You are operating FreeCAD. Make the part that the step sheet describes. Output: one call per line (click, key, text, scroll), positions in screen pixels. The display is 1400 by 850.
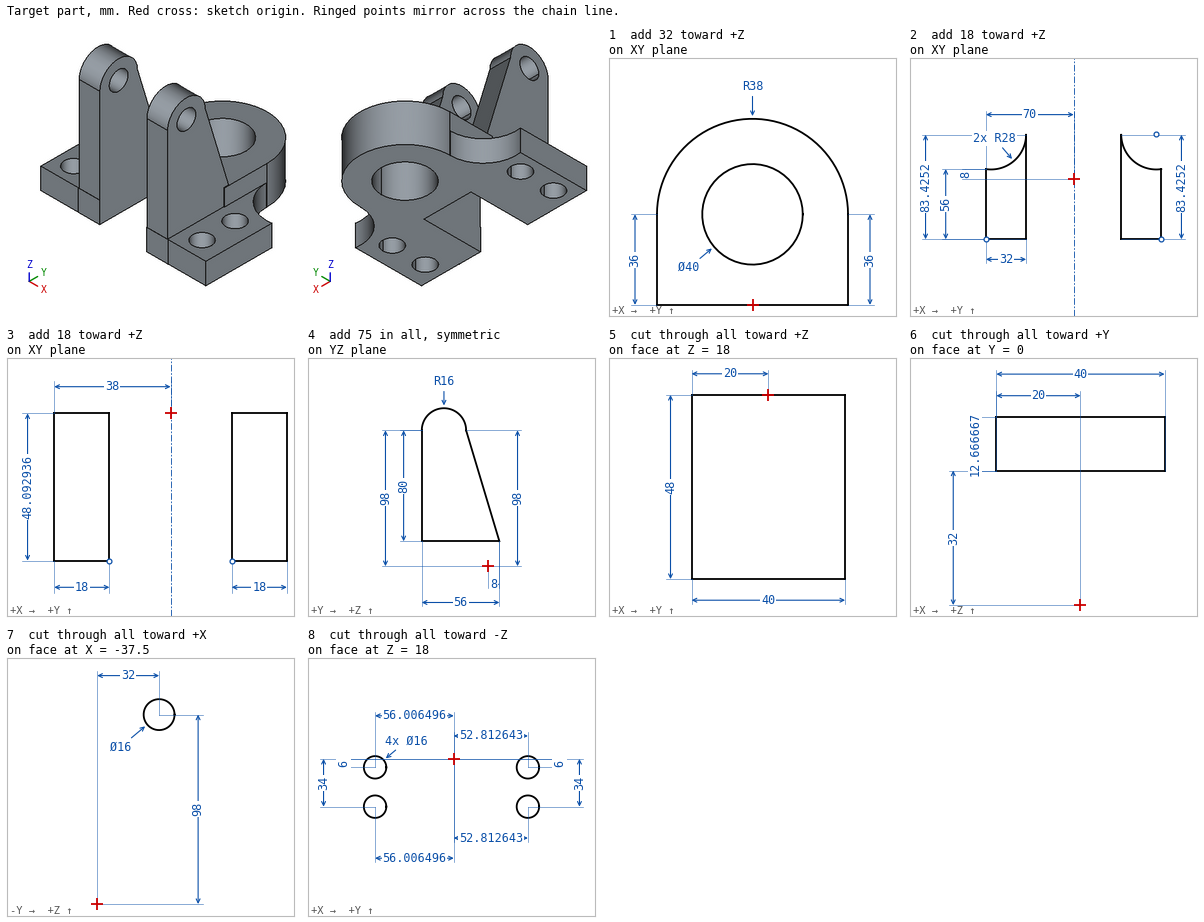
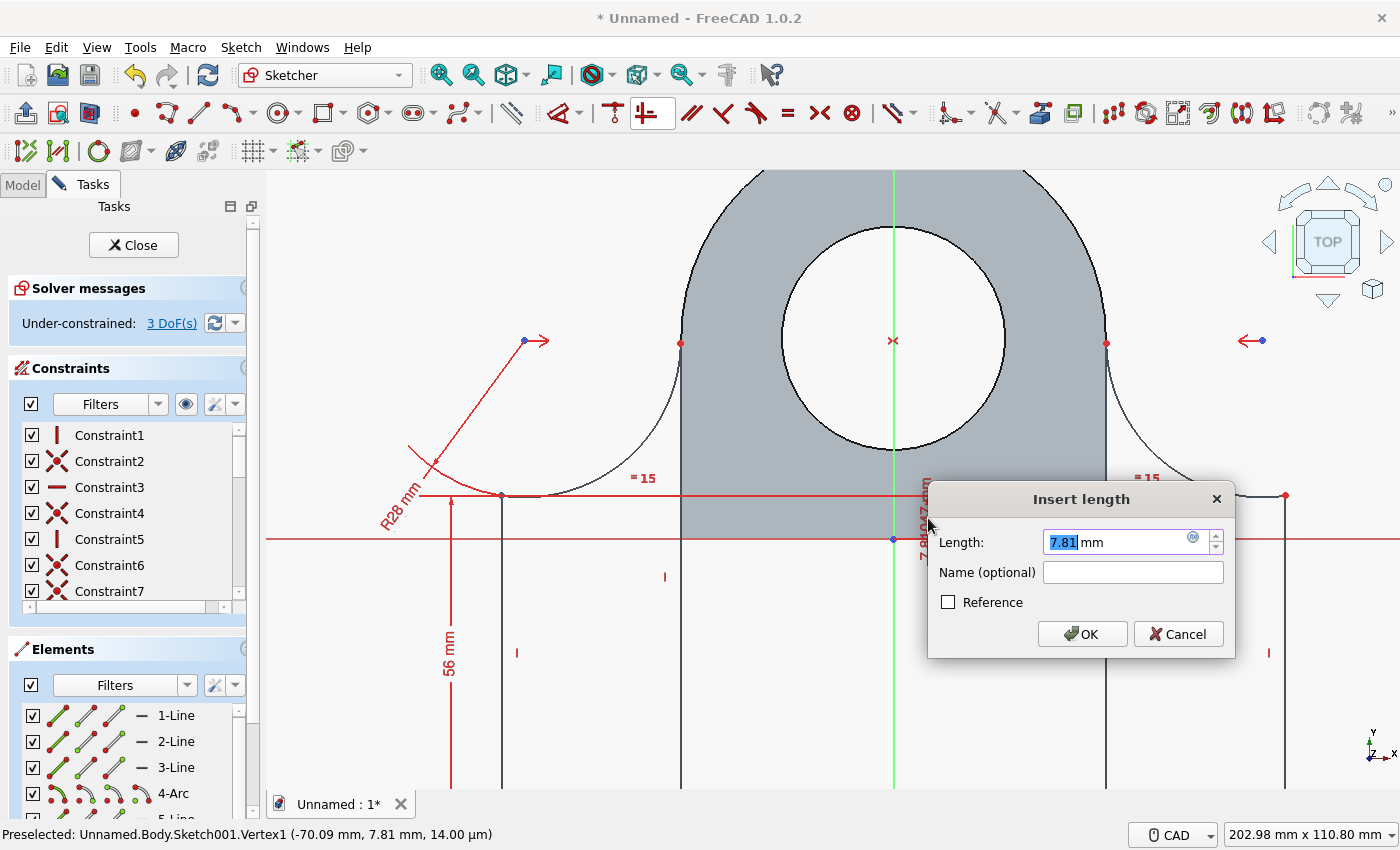
text(8)
key(Return)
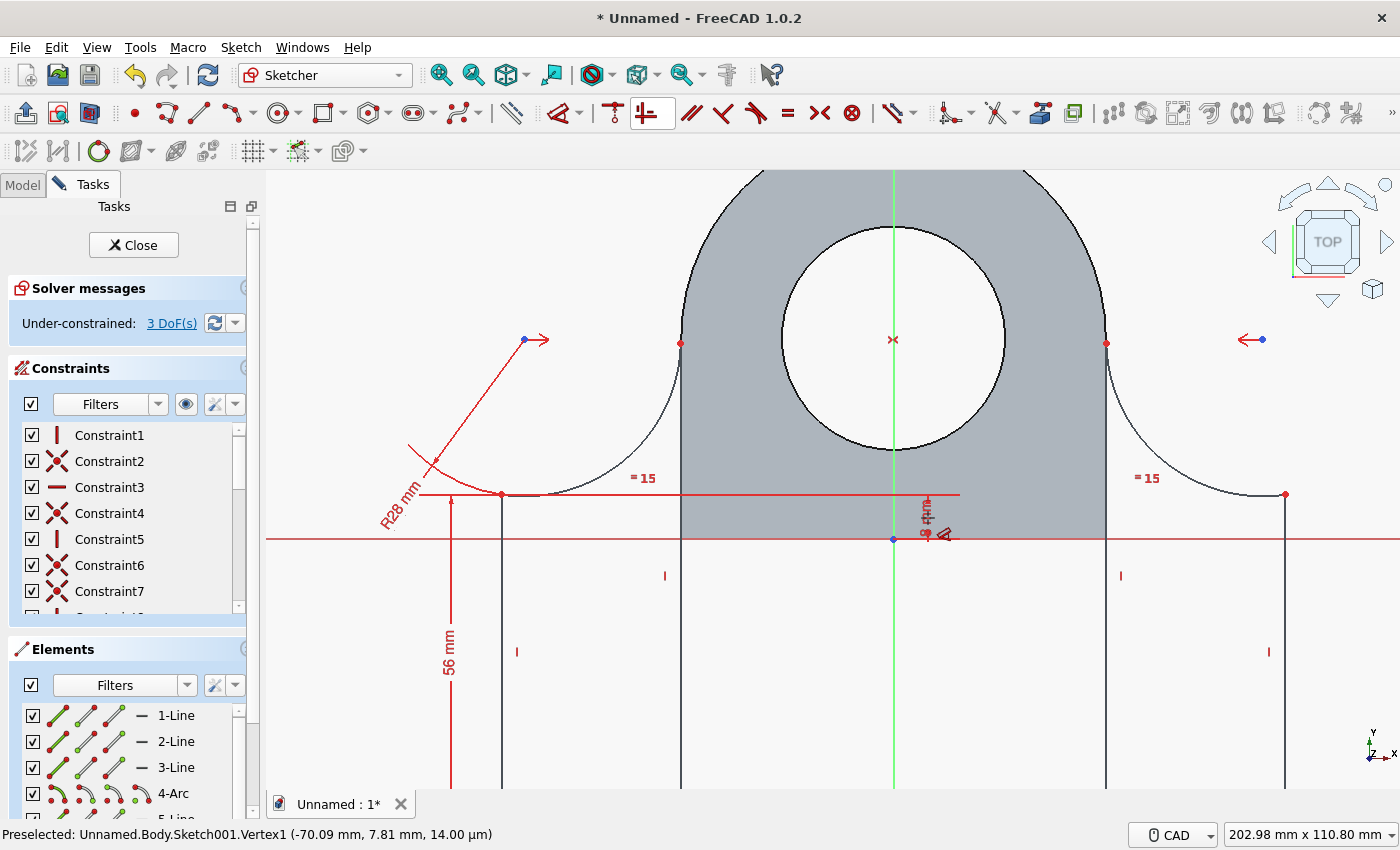
click(502, 495)
click(698, 461)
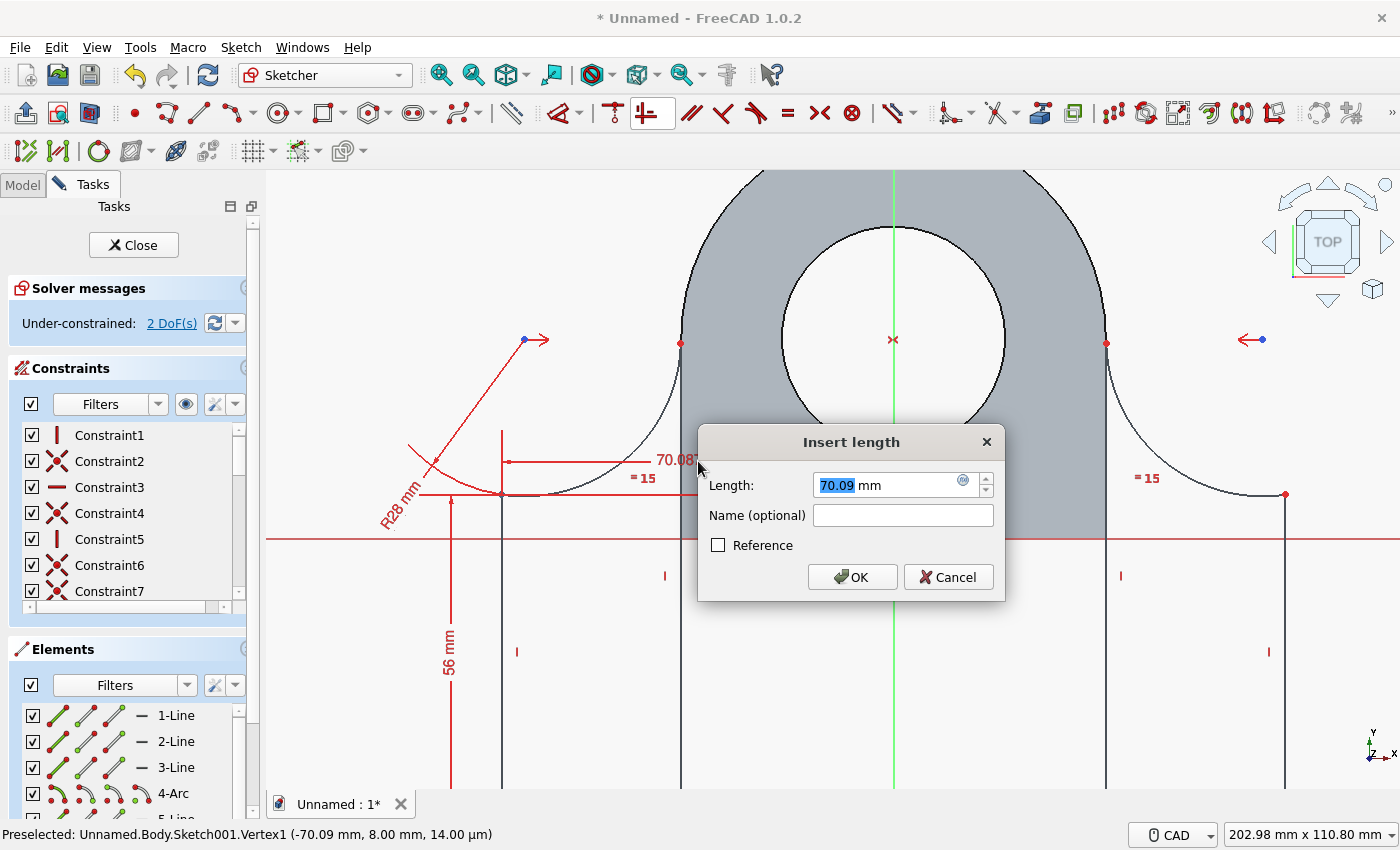
text(70)
key(Return)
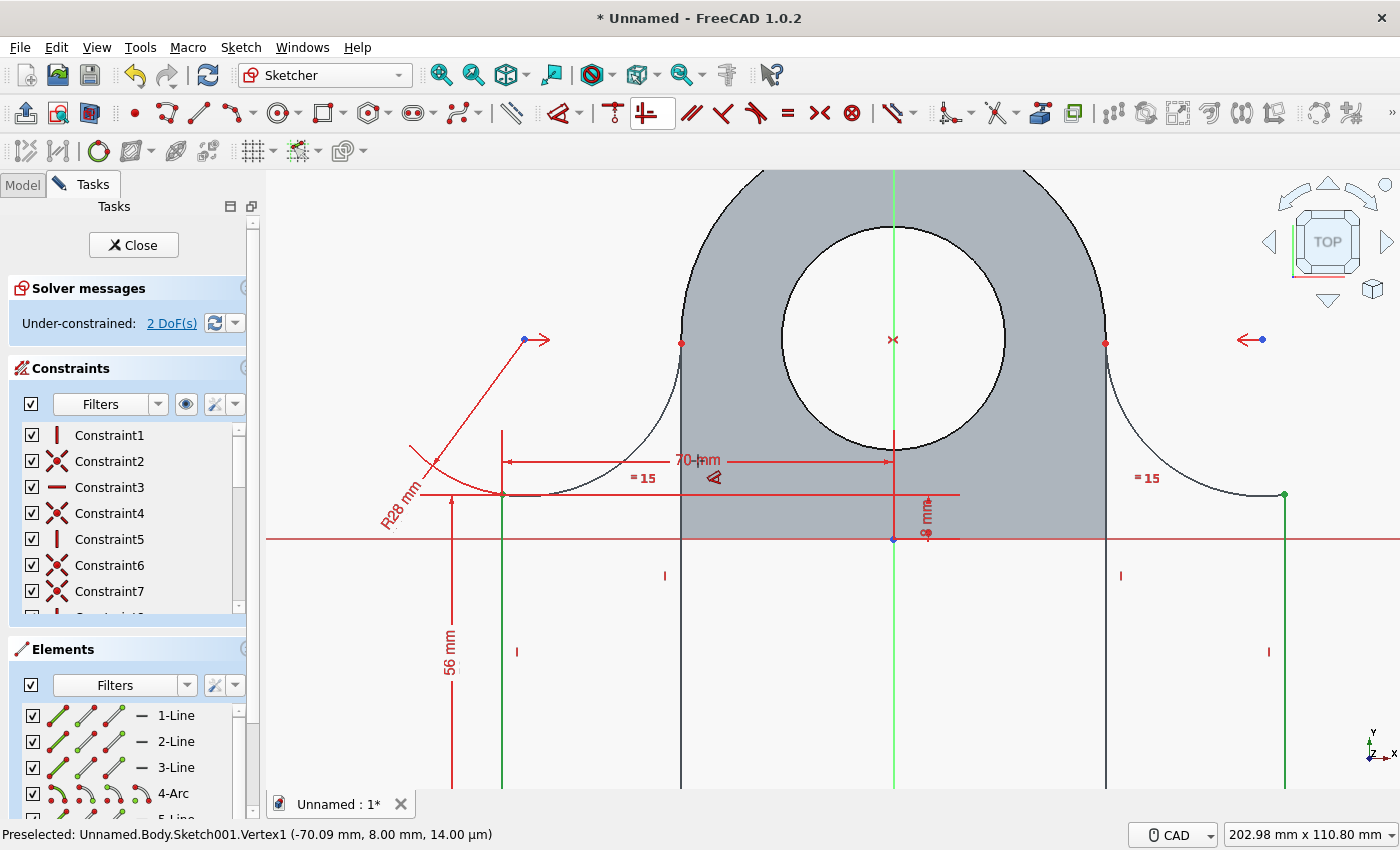
click(681, 668)
click(647, 648)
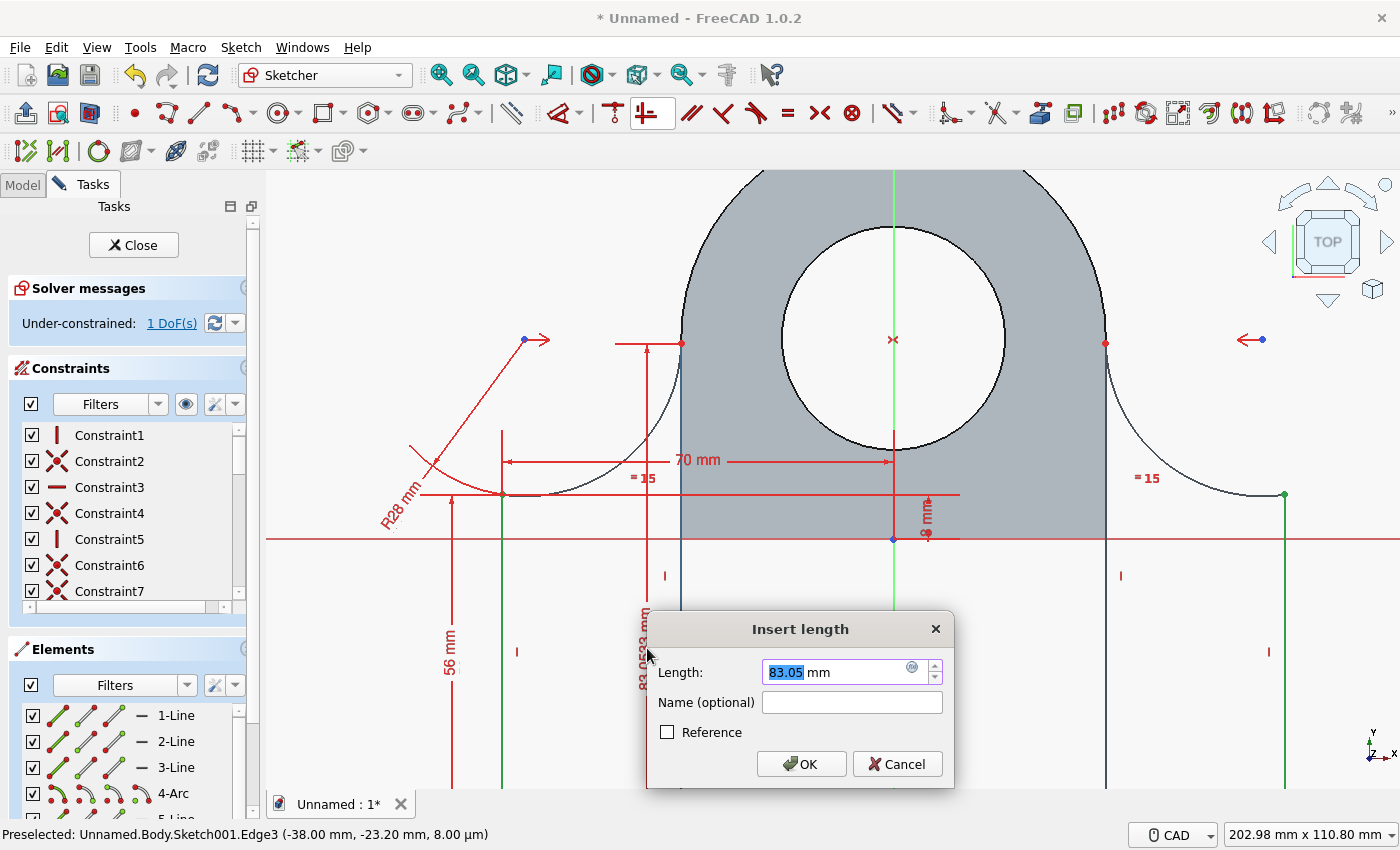
text(83.4252)
key(Return)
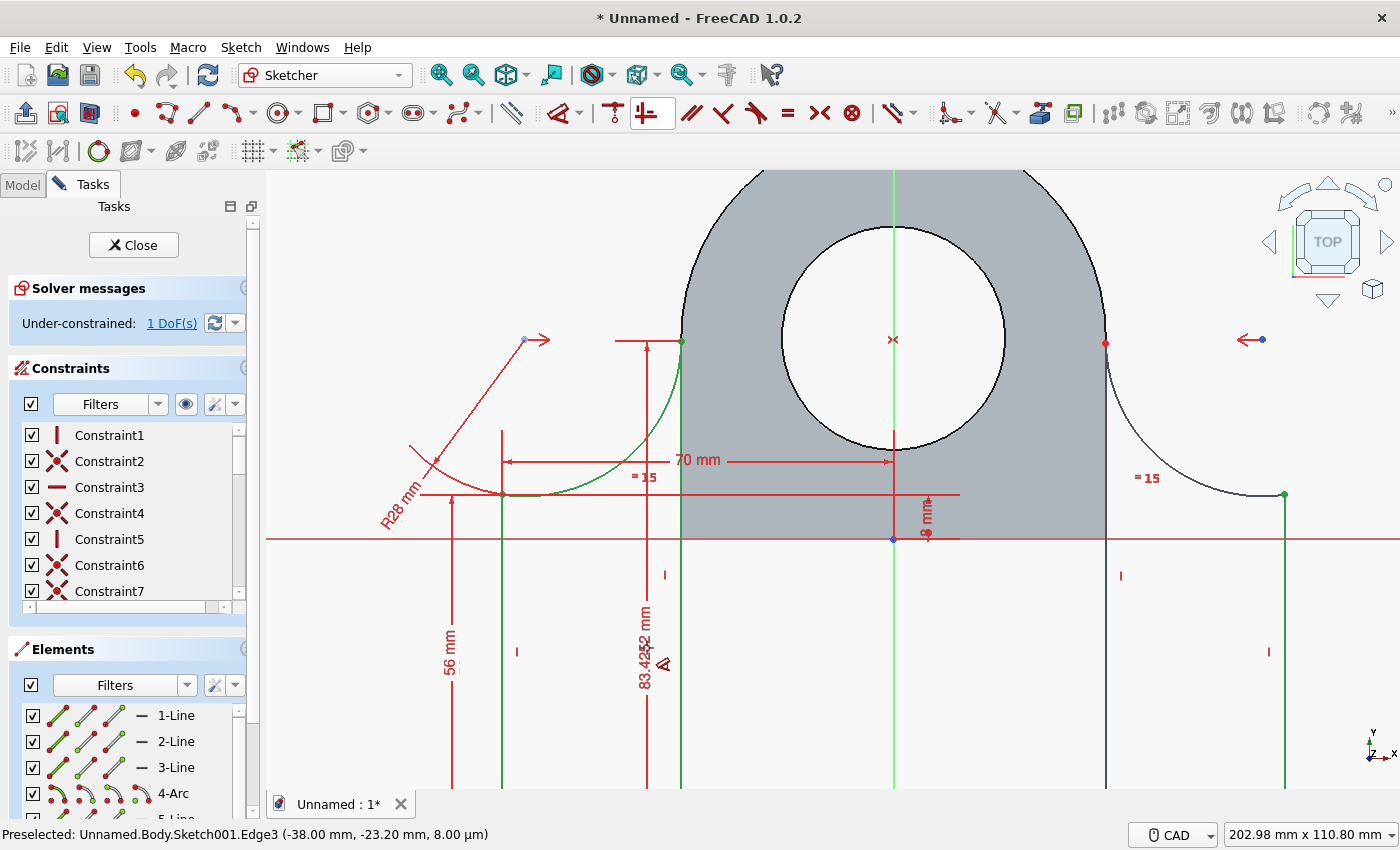
click(1106, 483)
click(1140, 648)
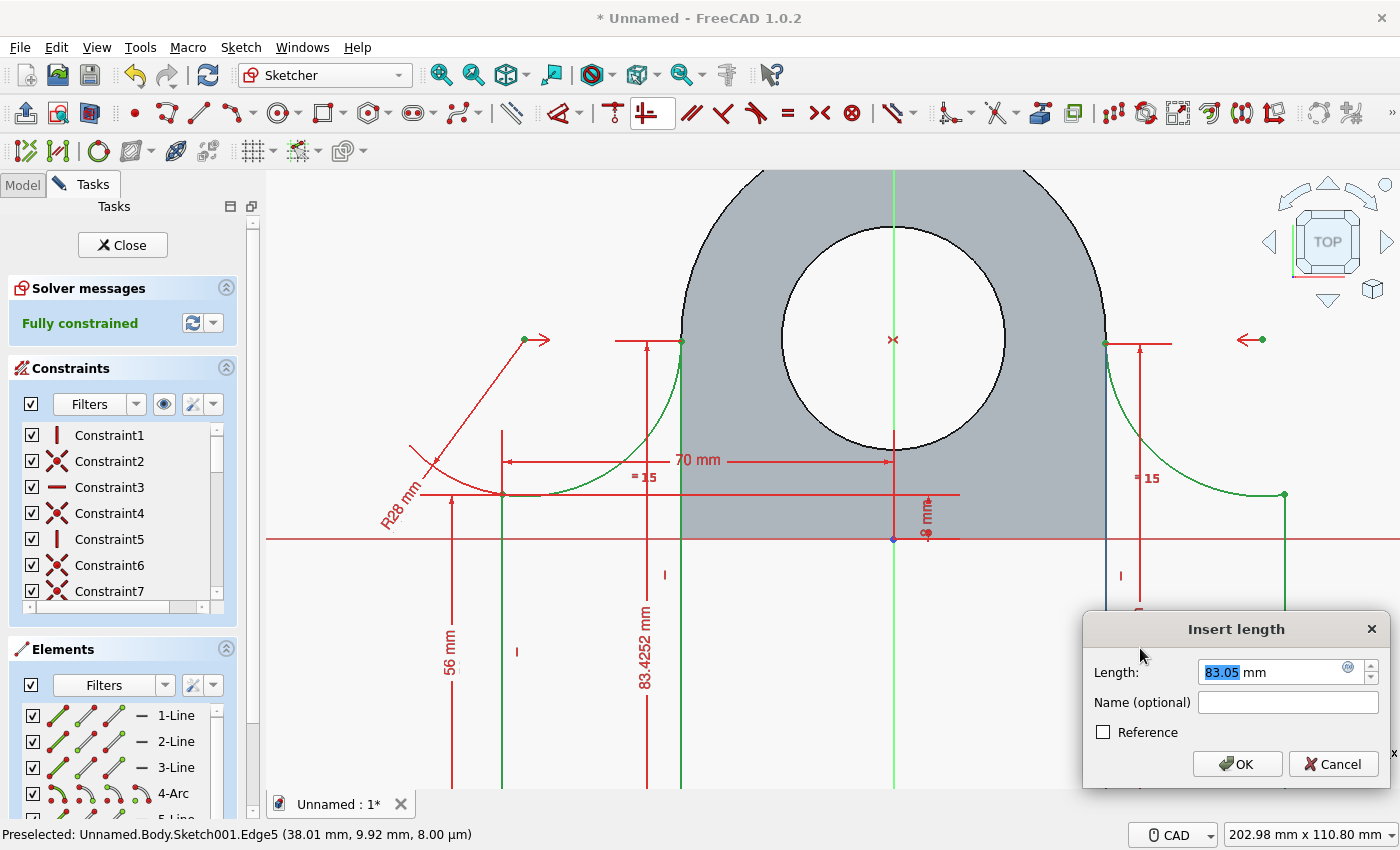
text(83.4252)
key(Return)
key(Escape)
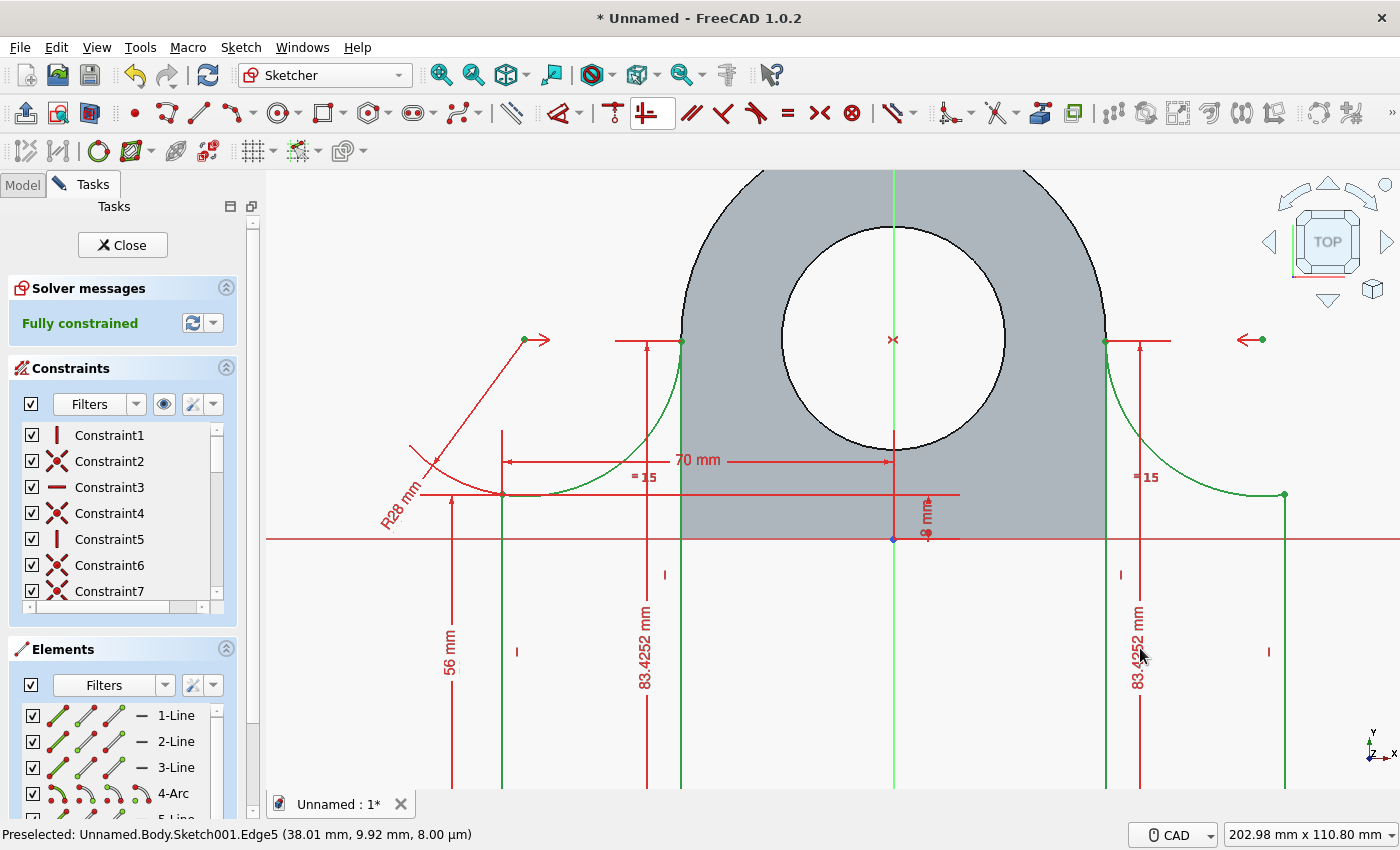
click(123, 245)